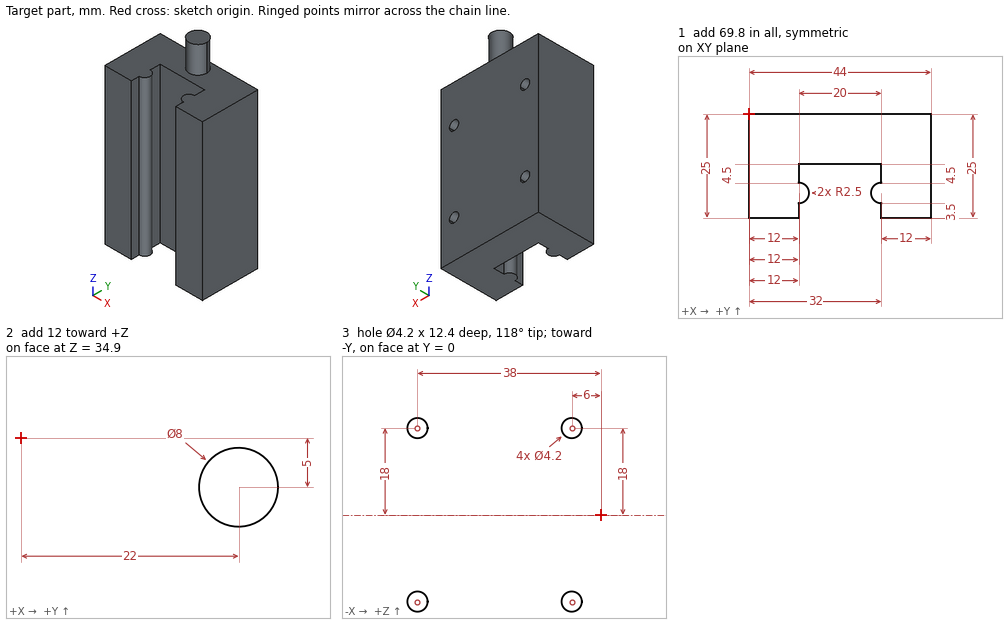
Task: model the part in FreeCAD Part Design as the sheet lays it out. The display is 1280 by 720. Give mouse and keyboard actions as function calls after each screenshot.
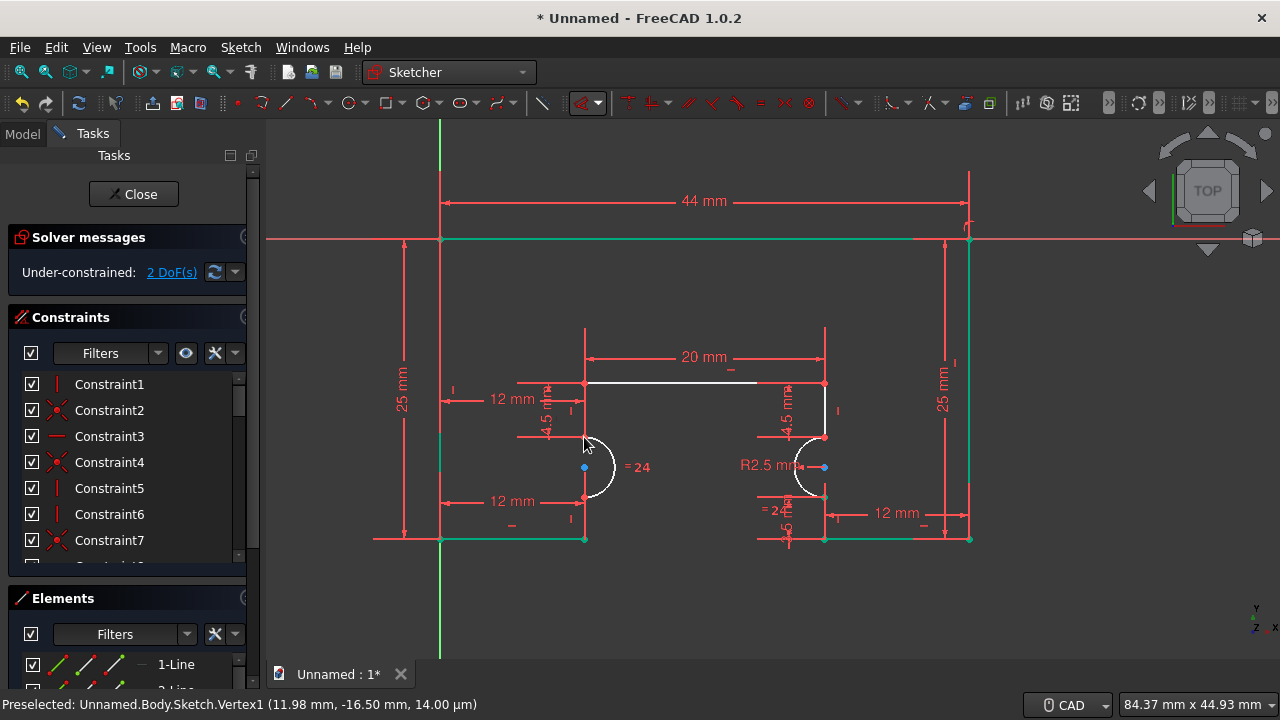
click(825, 467)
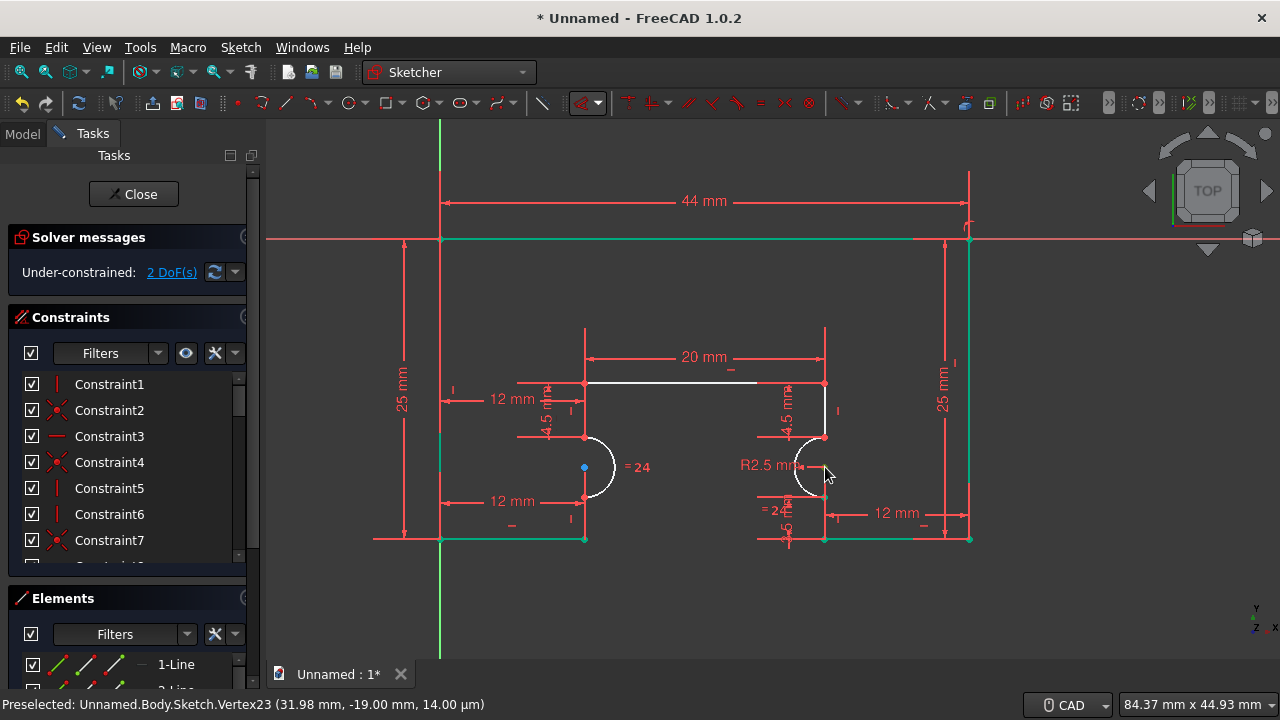
click(600, 104)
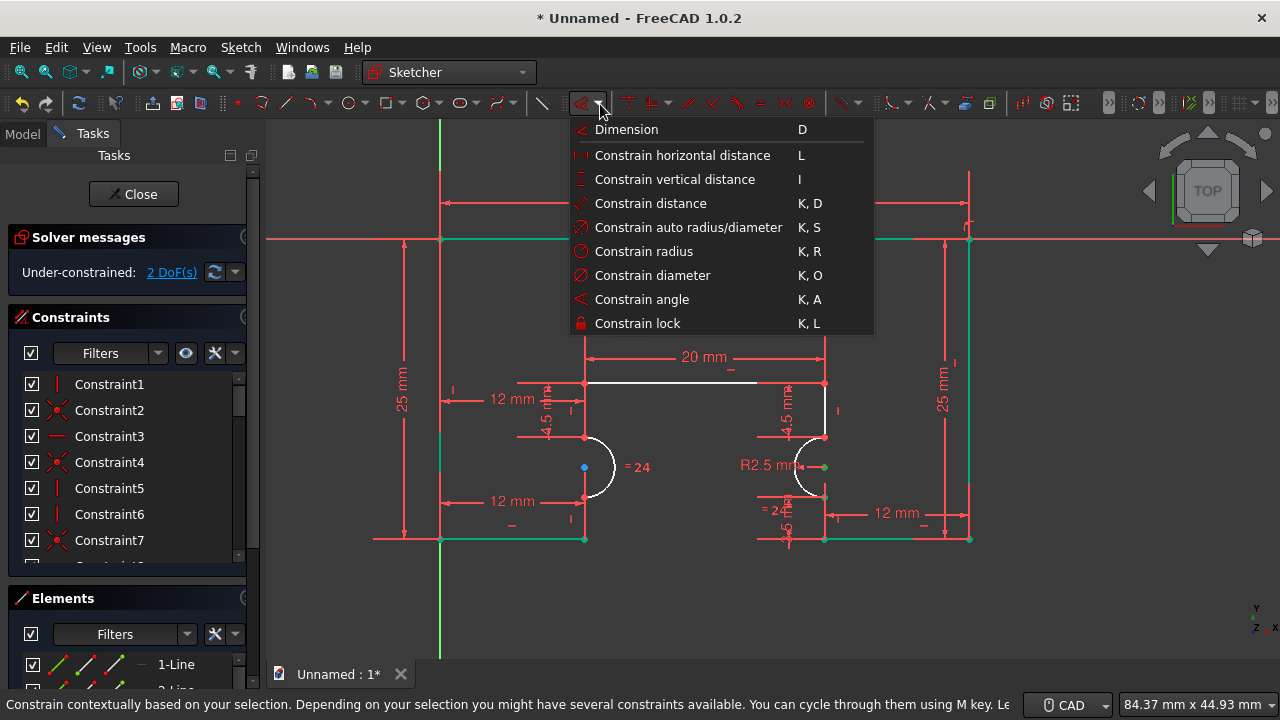
click(722, 155)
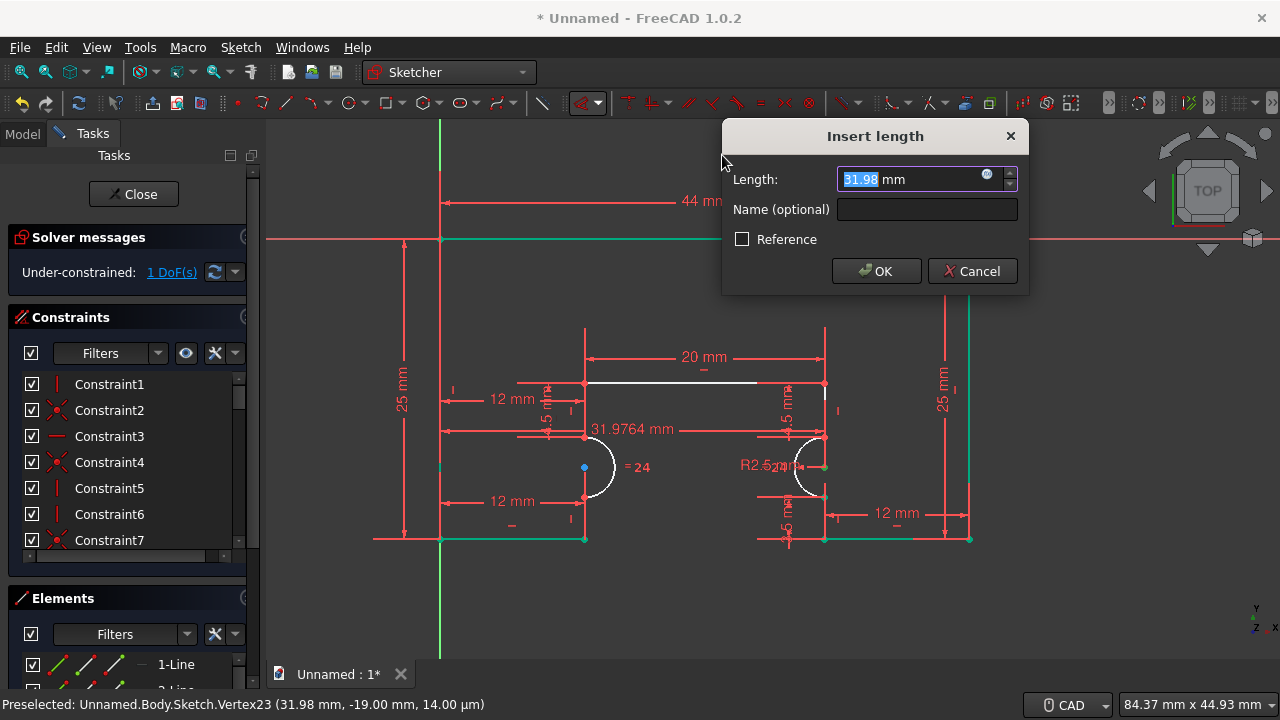
text(32)
key(Return)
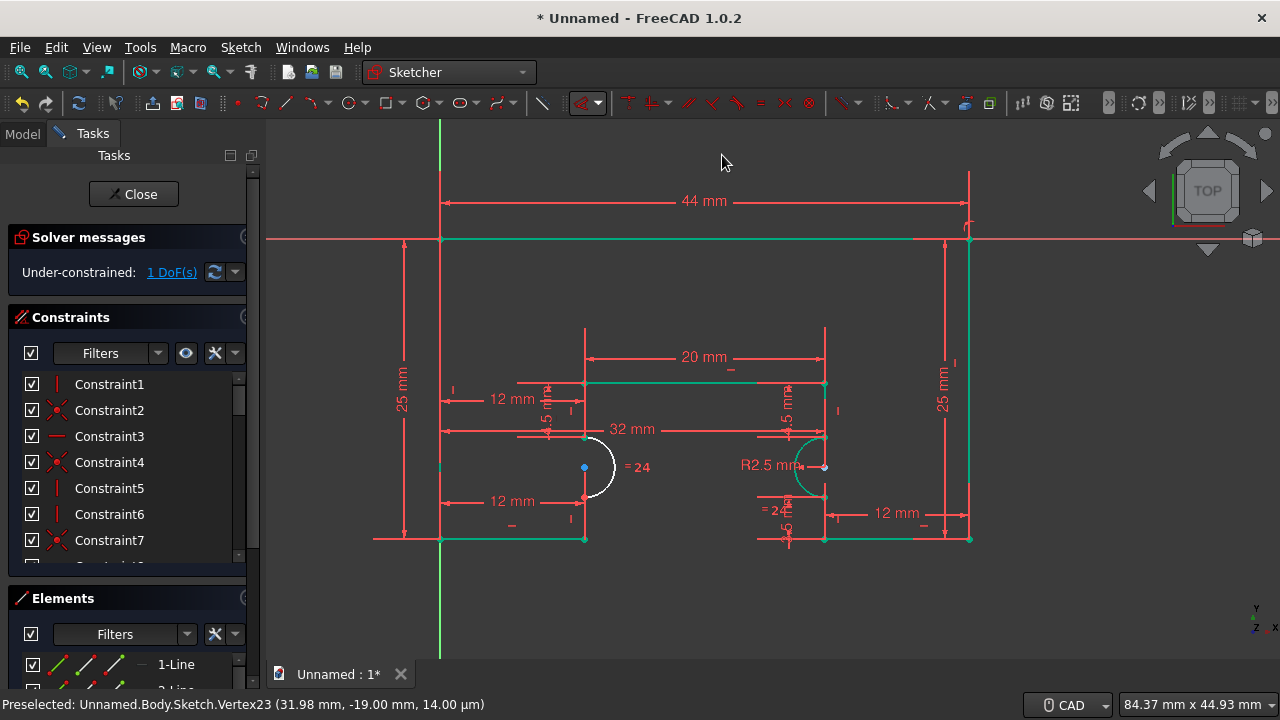
click(585, 467)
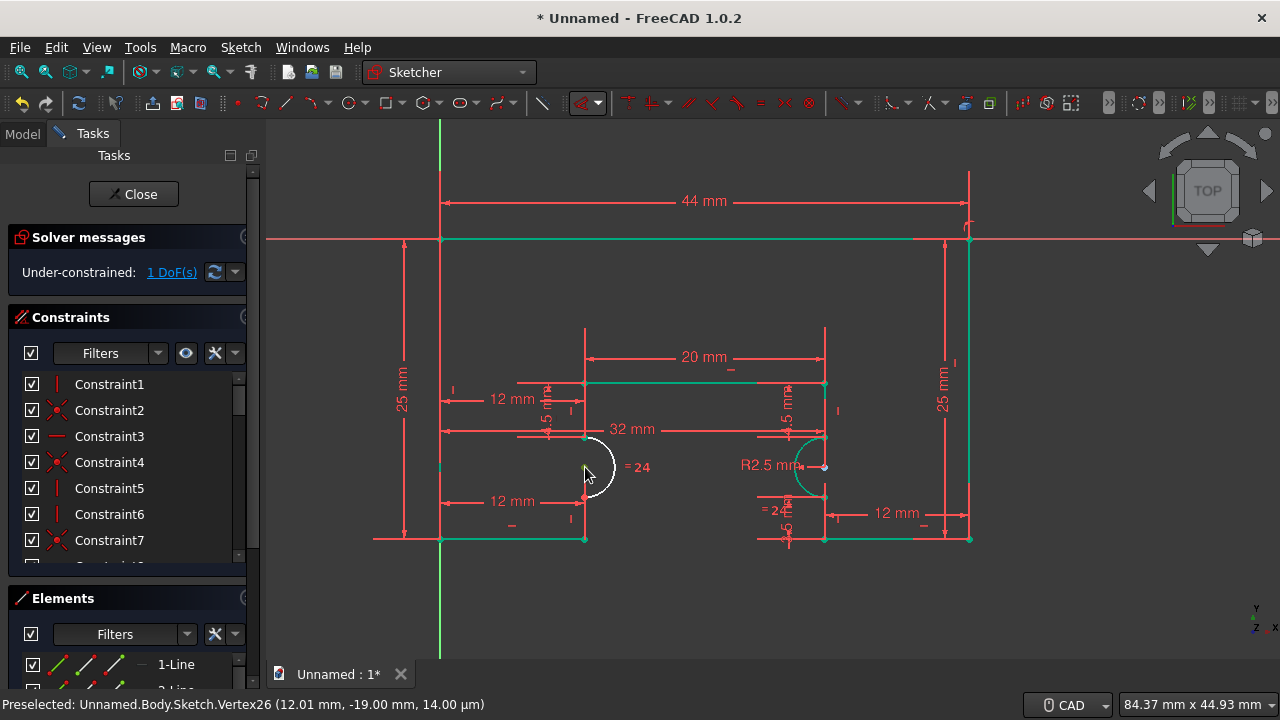
key(l)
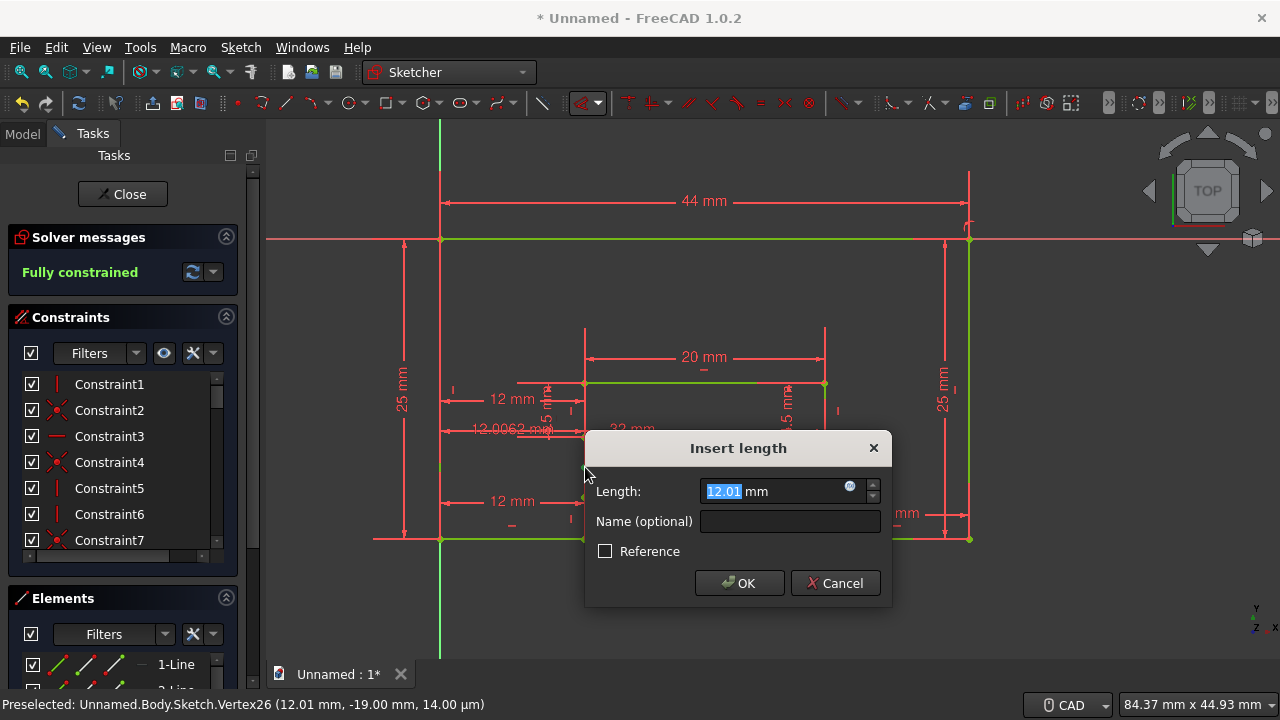
text(12)
key(Return)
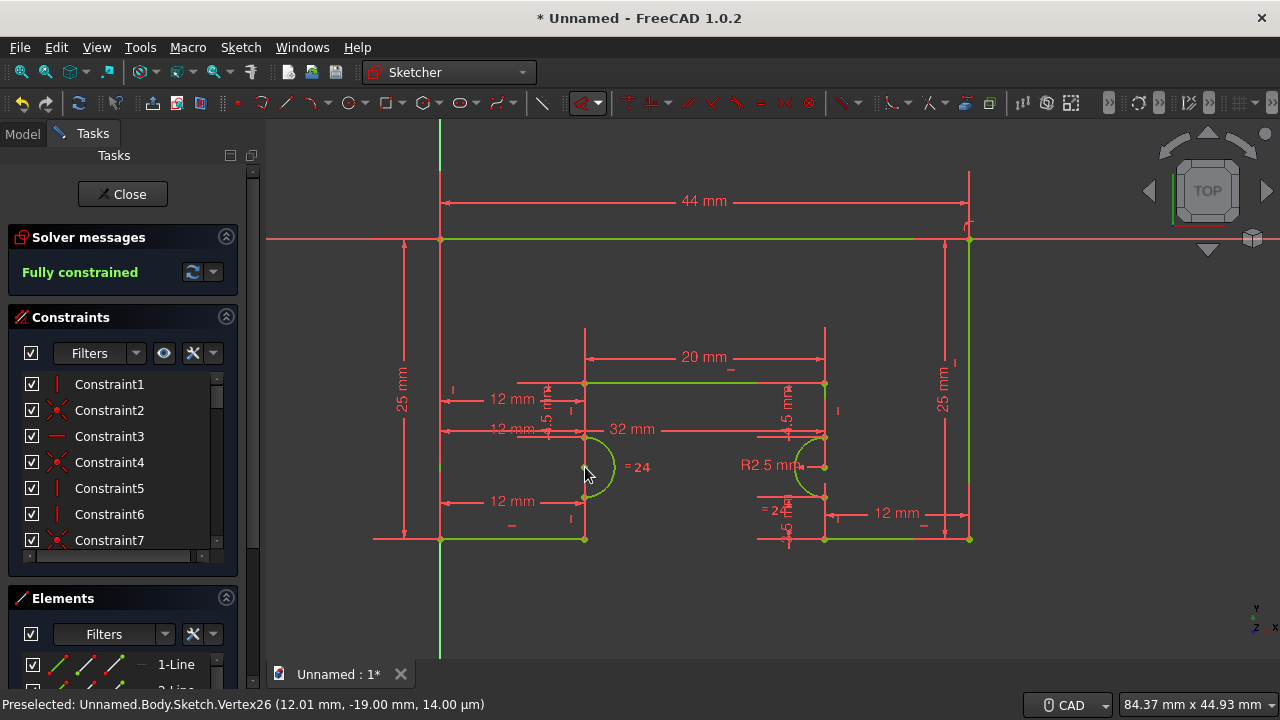
click(123, 194)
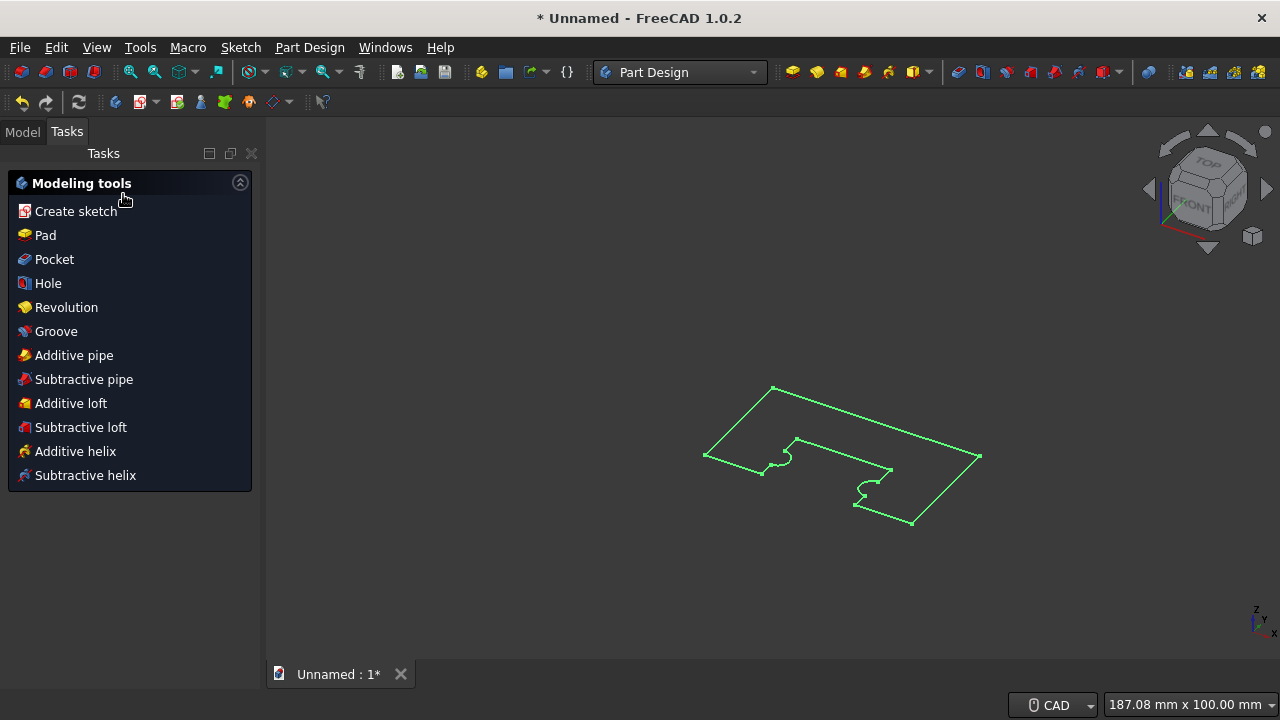
click(794, 72)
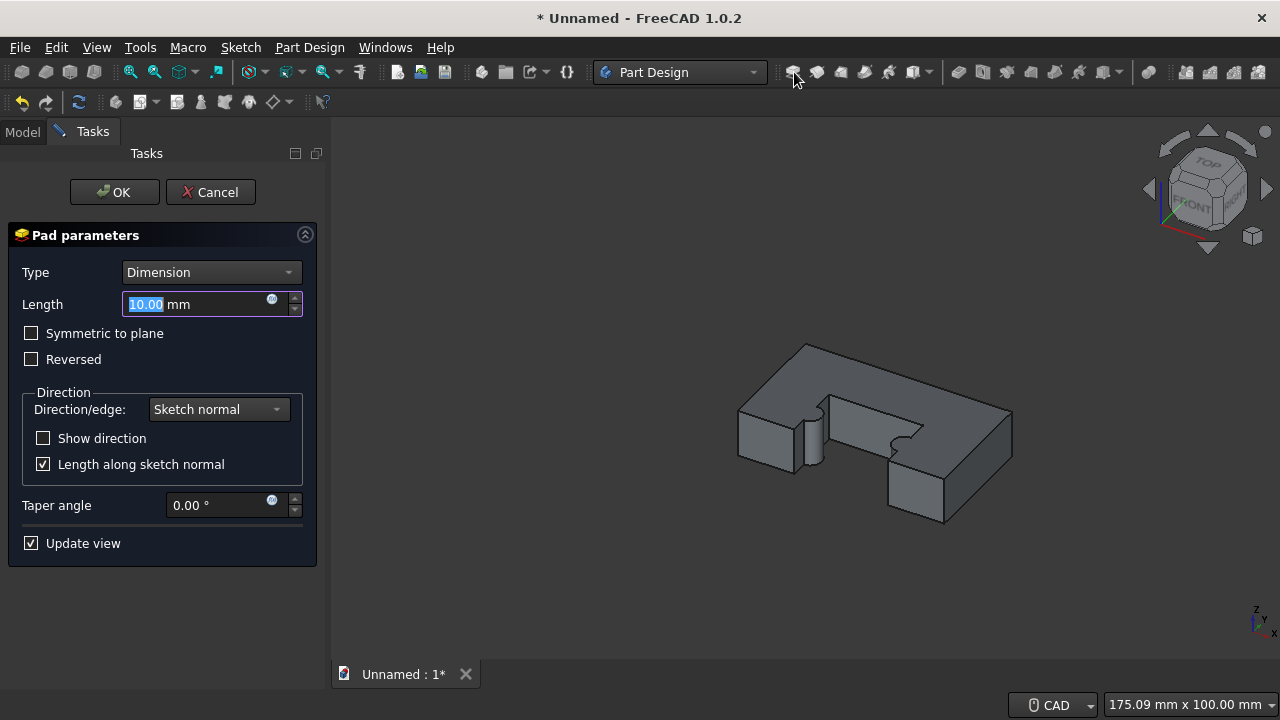
text(69.8)
key(Tab)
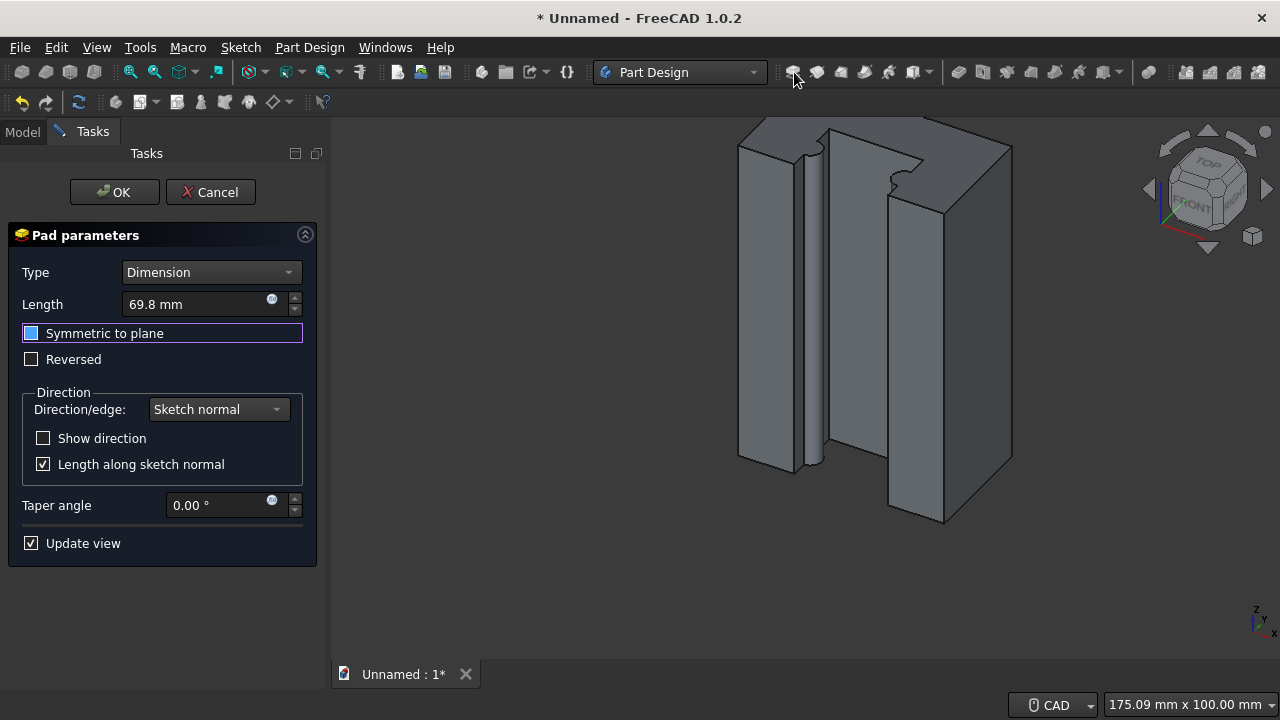
click(30, 333)